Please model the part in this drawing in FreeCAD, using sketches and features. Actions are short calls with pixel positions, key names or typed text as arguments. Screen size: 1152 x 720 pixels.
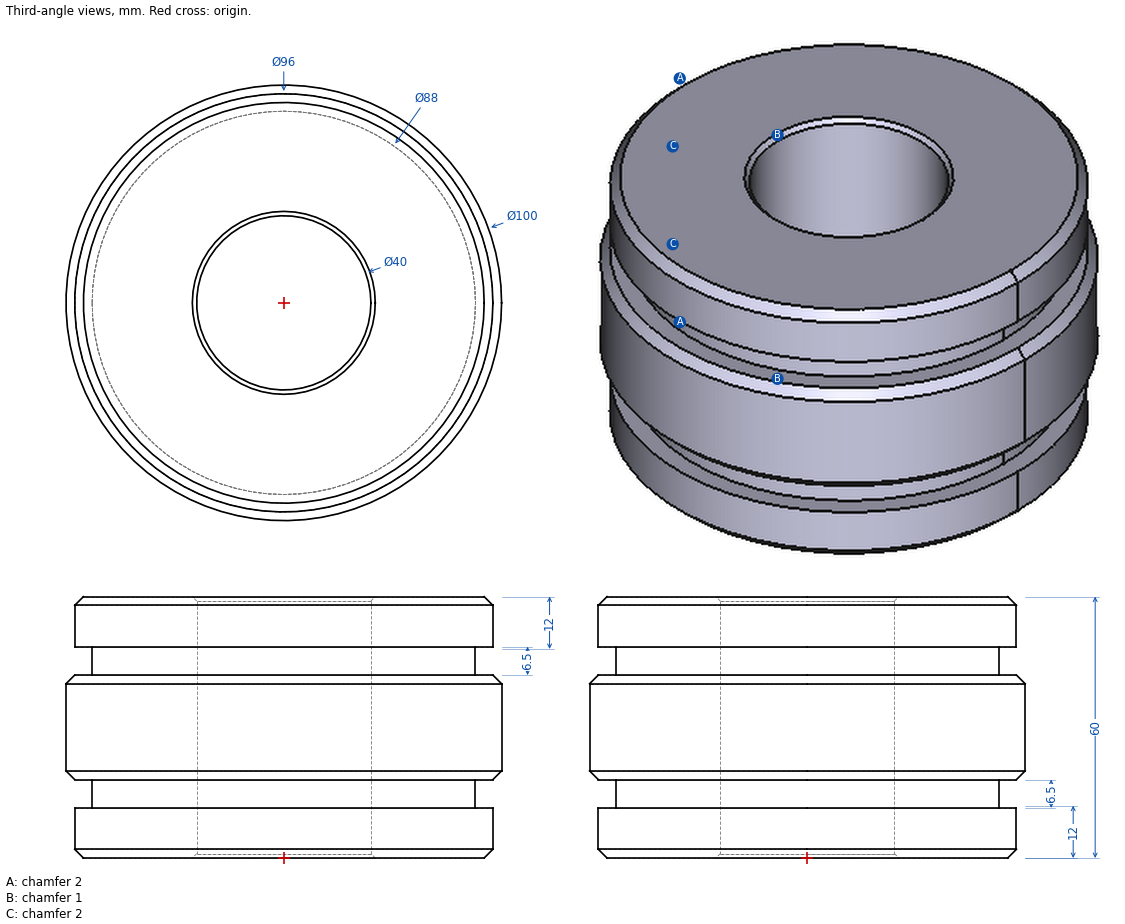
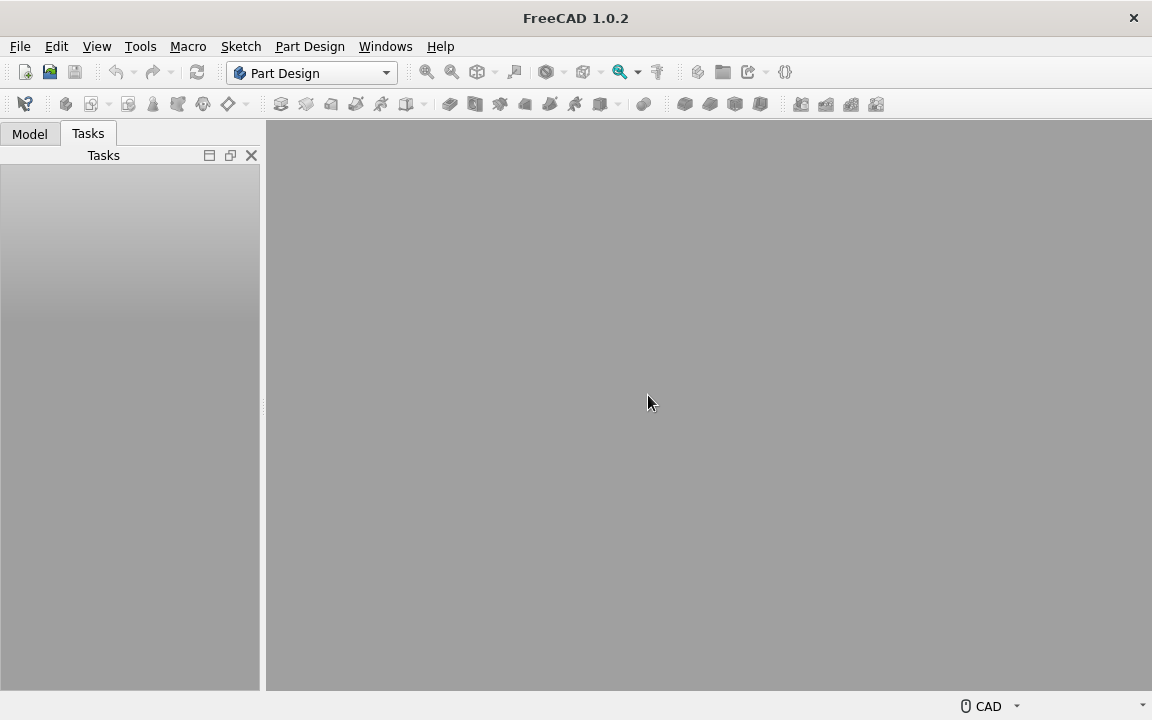
click(25, 72)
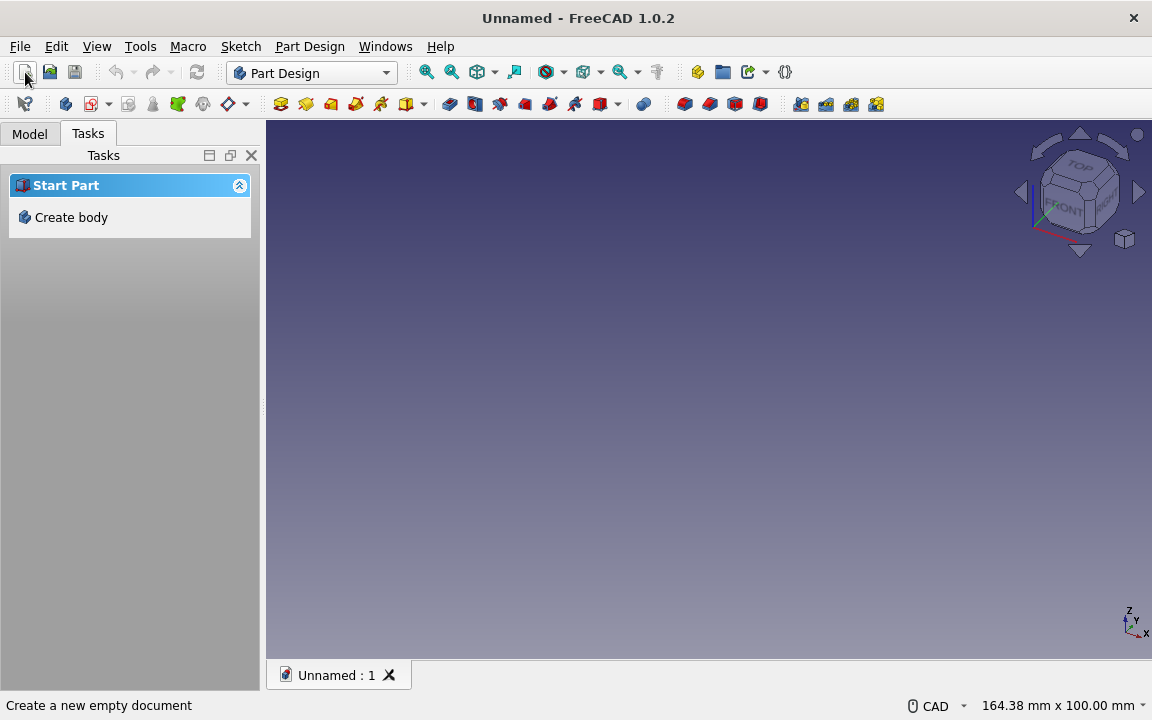
click(90, 104)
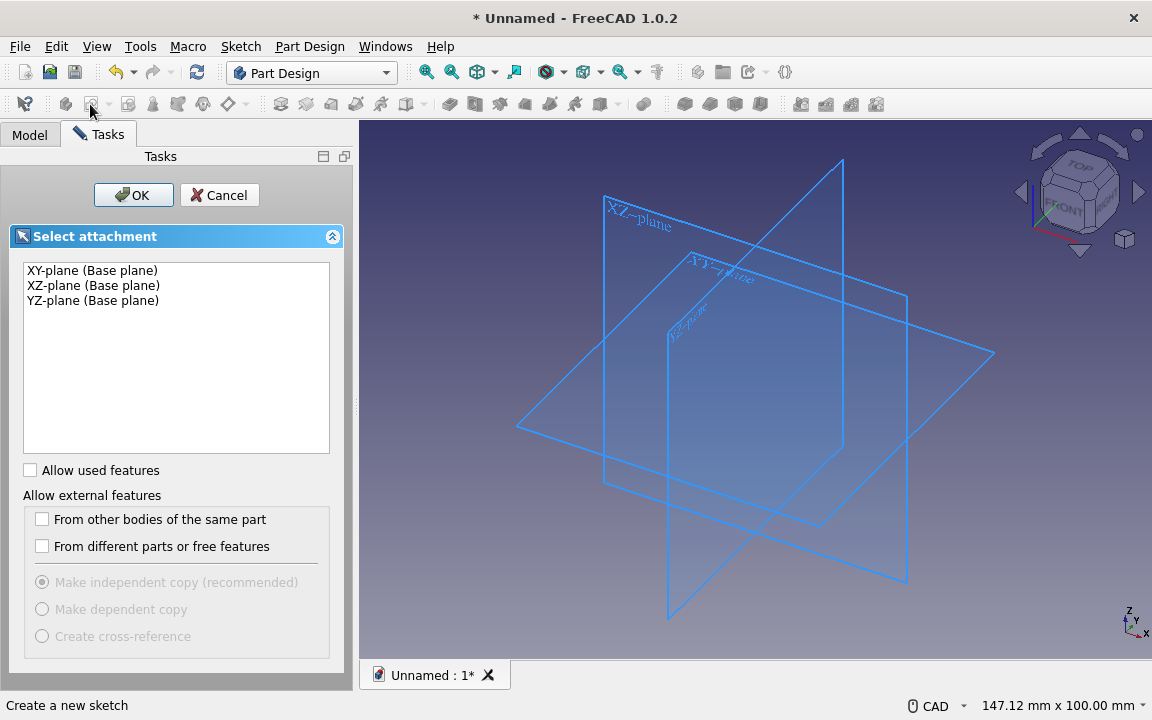
click(84, 270)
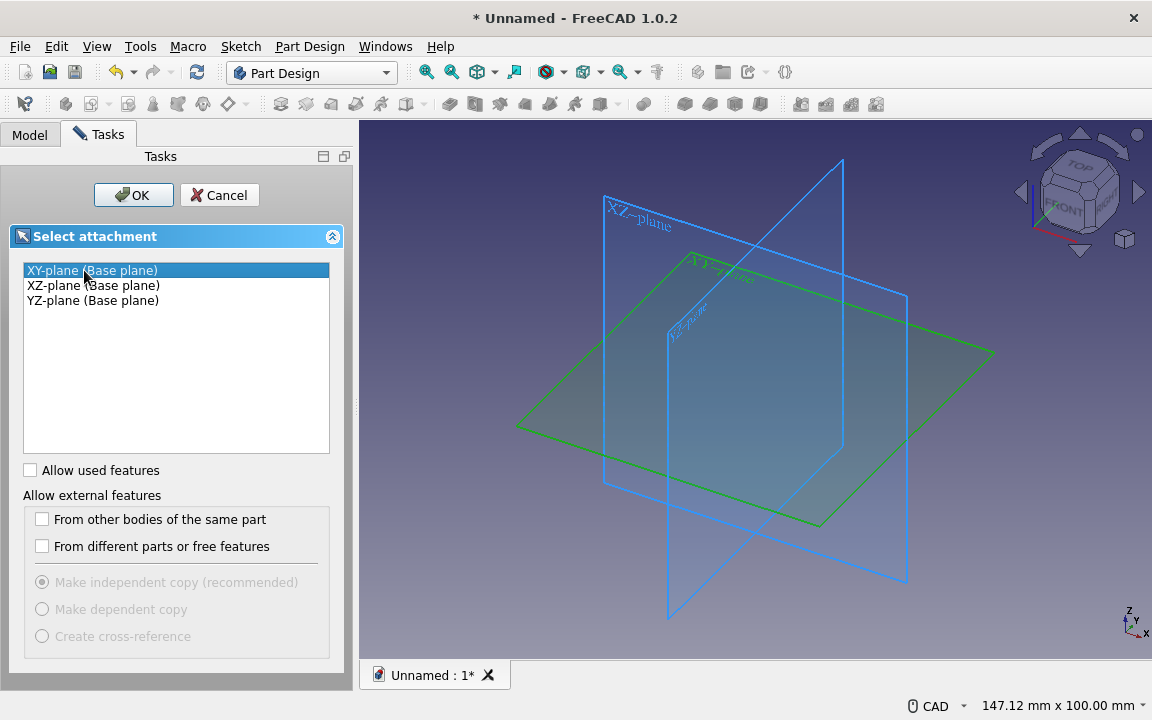
click(134, 195)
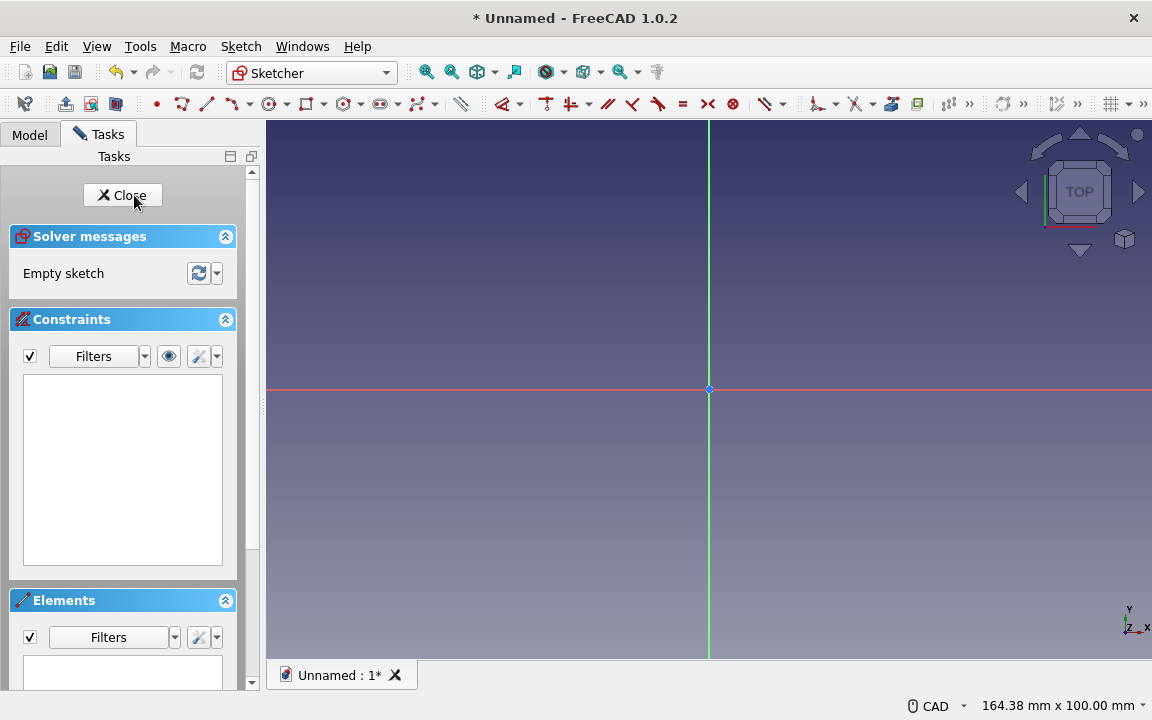
scroll(501, 390, down, 2)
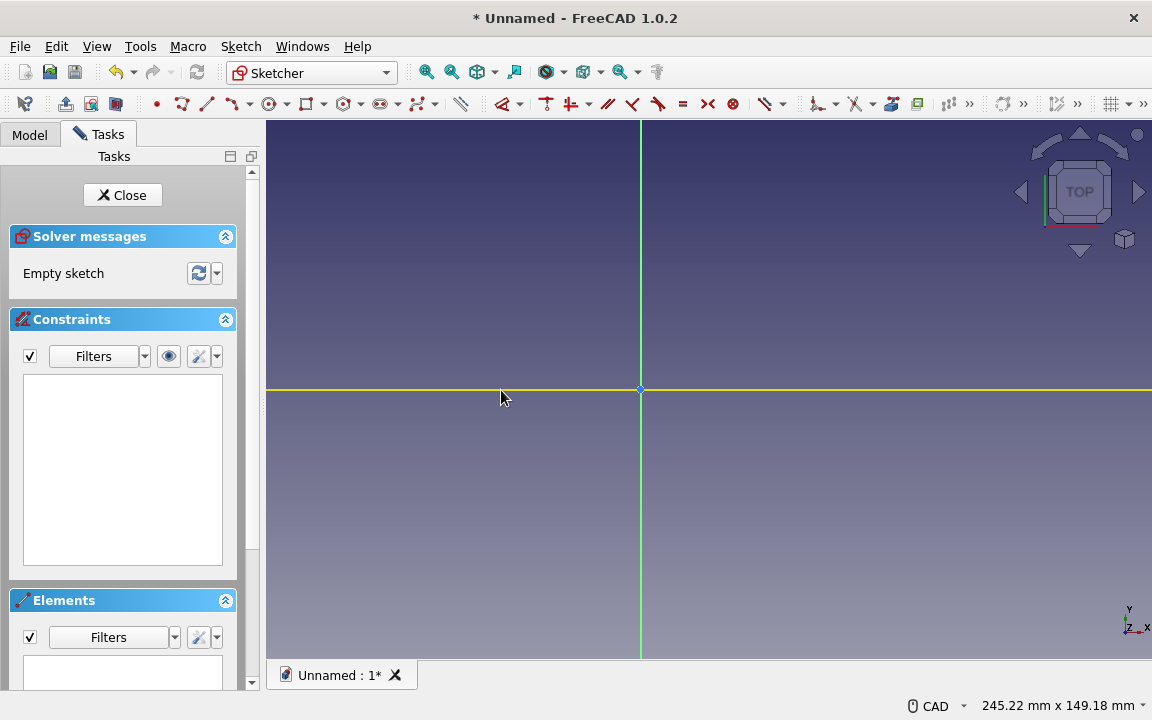
click(268, 104)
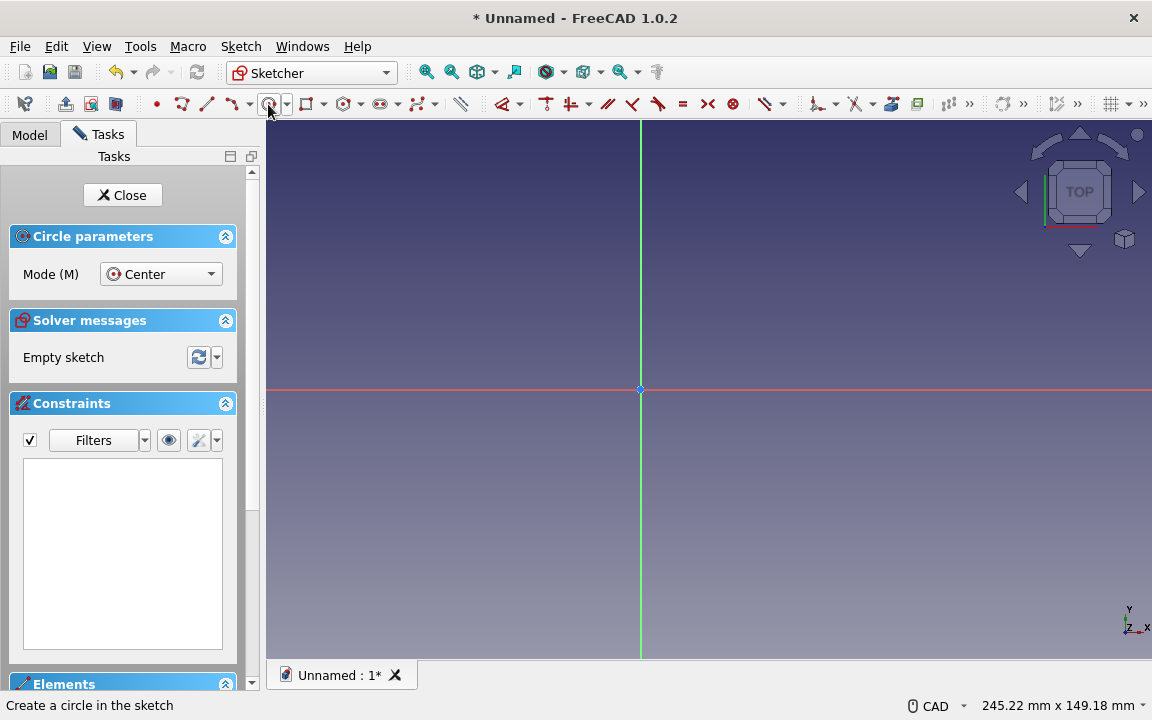
click(641, 390)
click(768, 262)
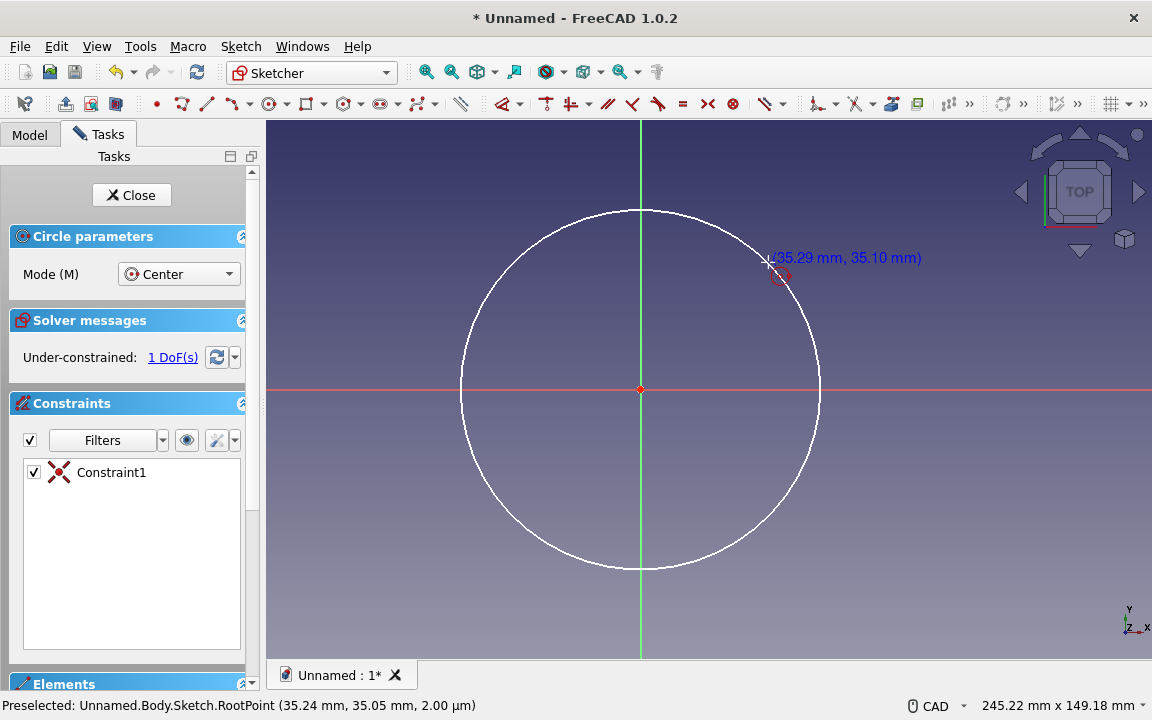
click(641, 390)
click(692, 339)
key(Escape)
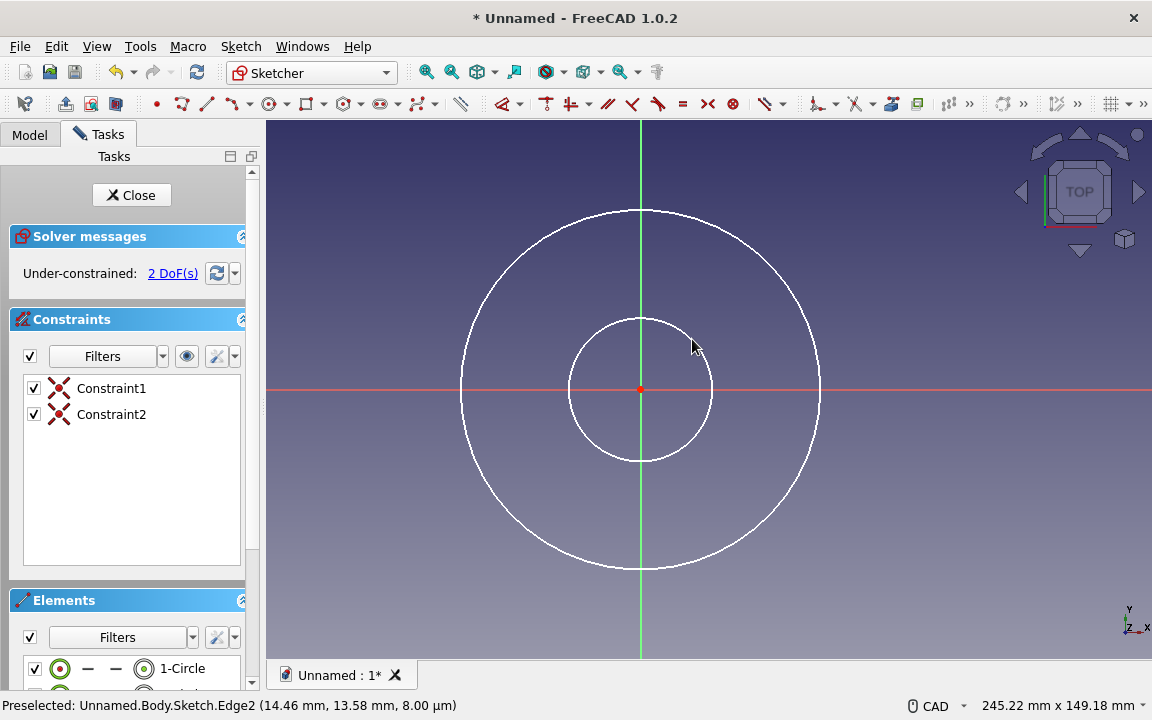
click(502, 104)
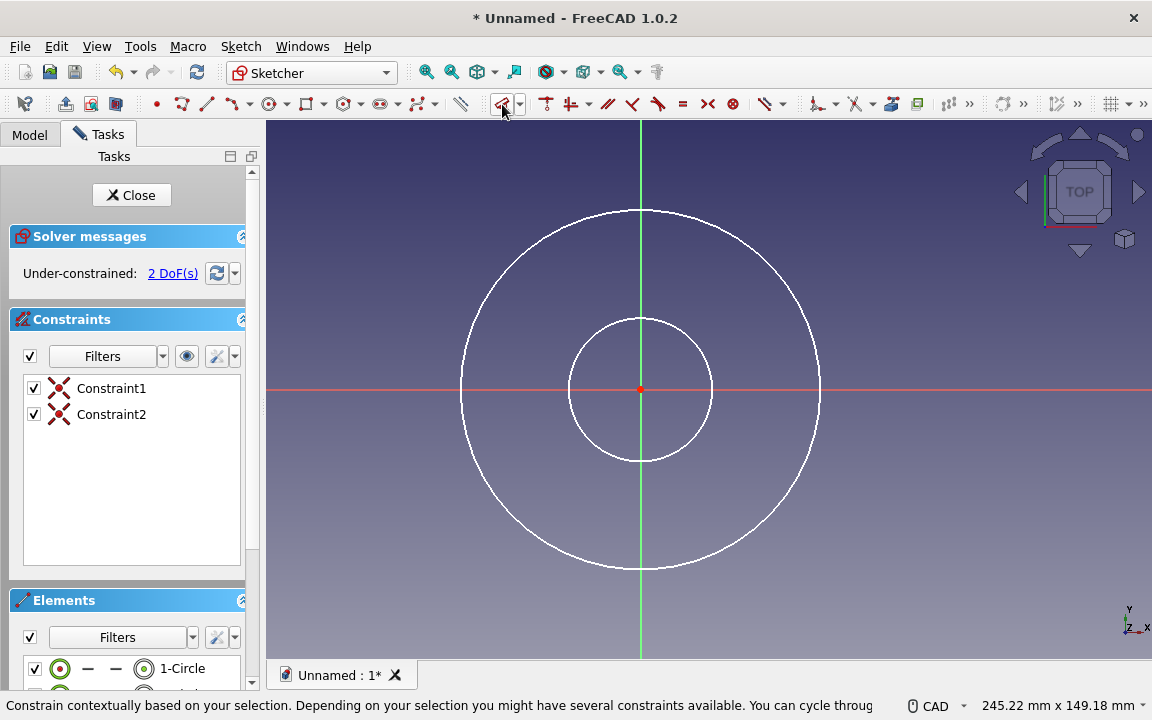
click(767, 262)
click(790, 239)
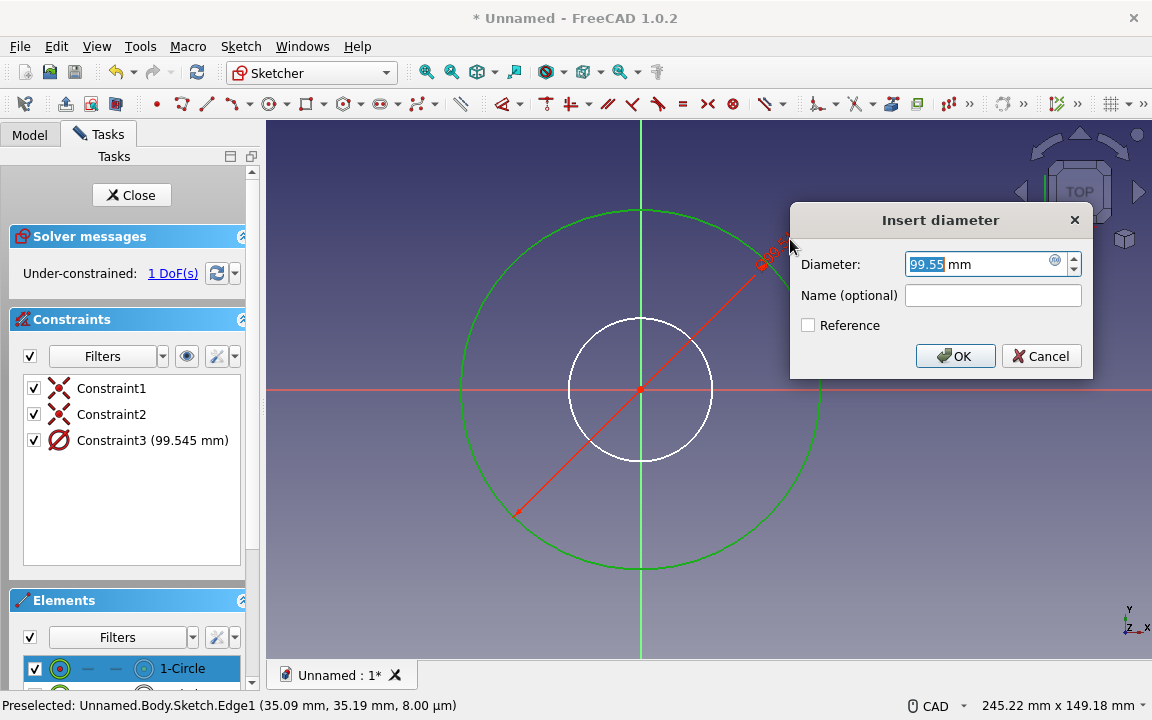
text(100)
key(Return)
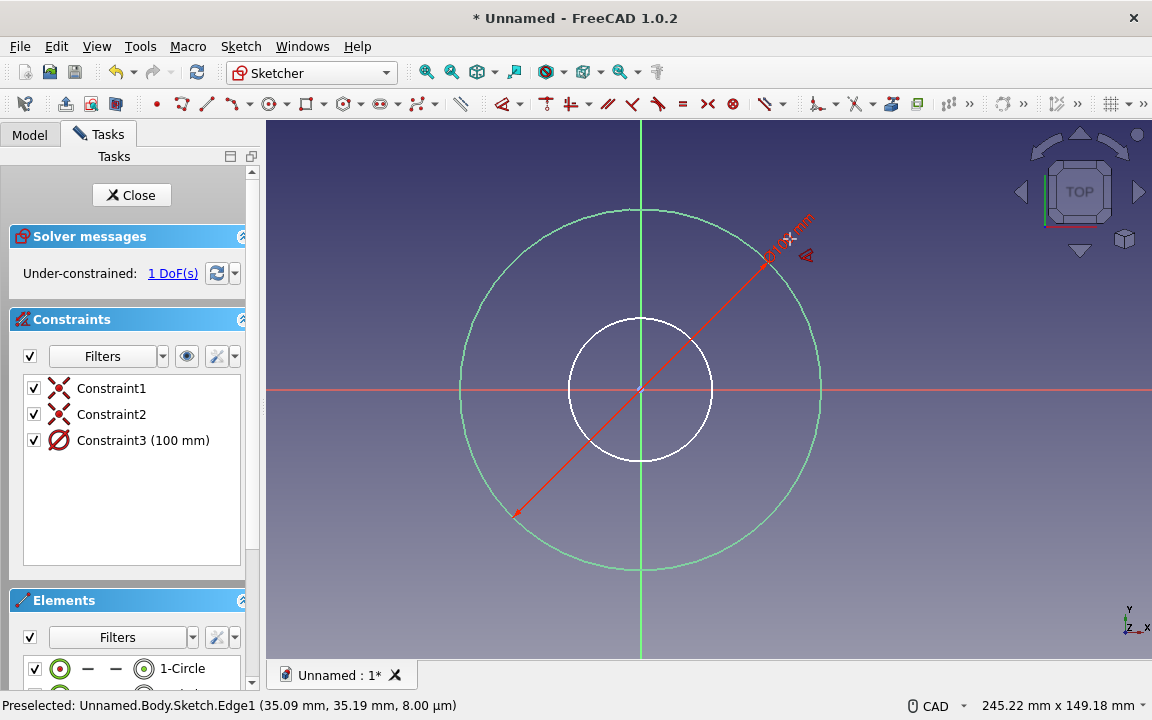
click(691, 339)
click(714, 316)